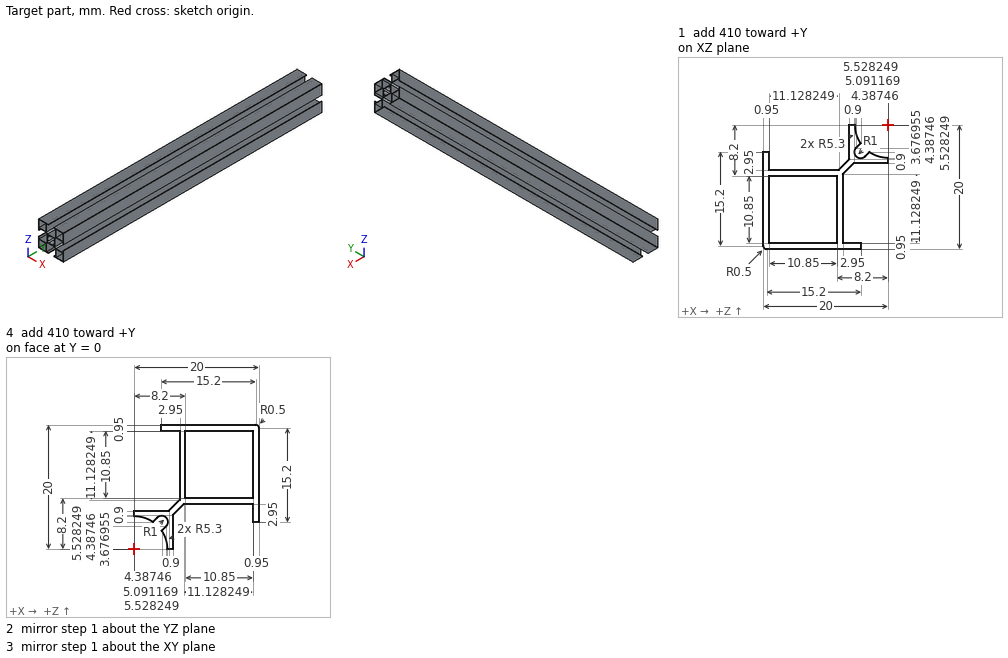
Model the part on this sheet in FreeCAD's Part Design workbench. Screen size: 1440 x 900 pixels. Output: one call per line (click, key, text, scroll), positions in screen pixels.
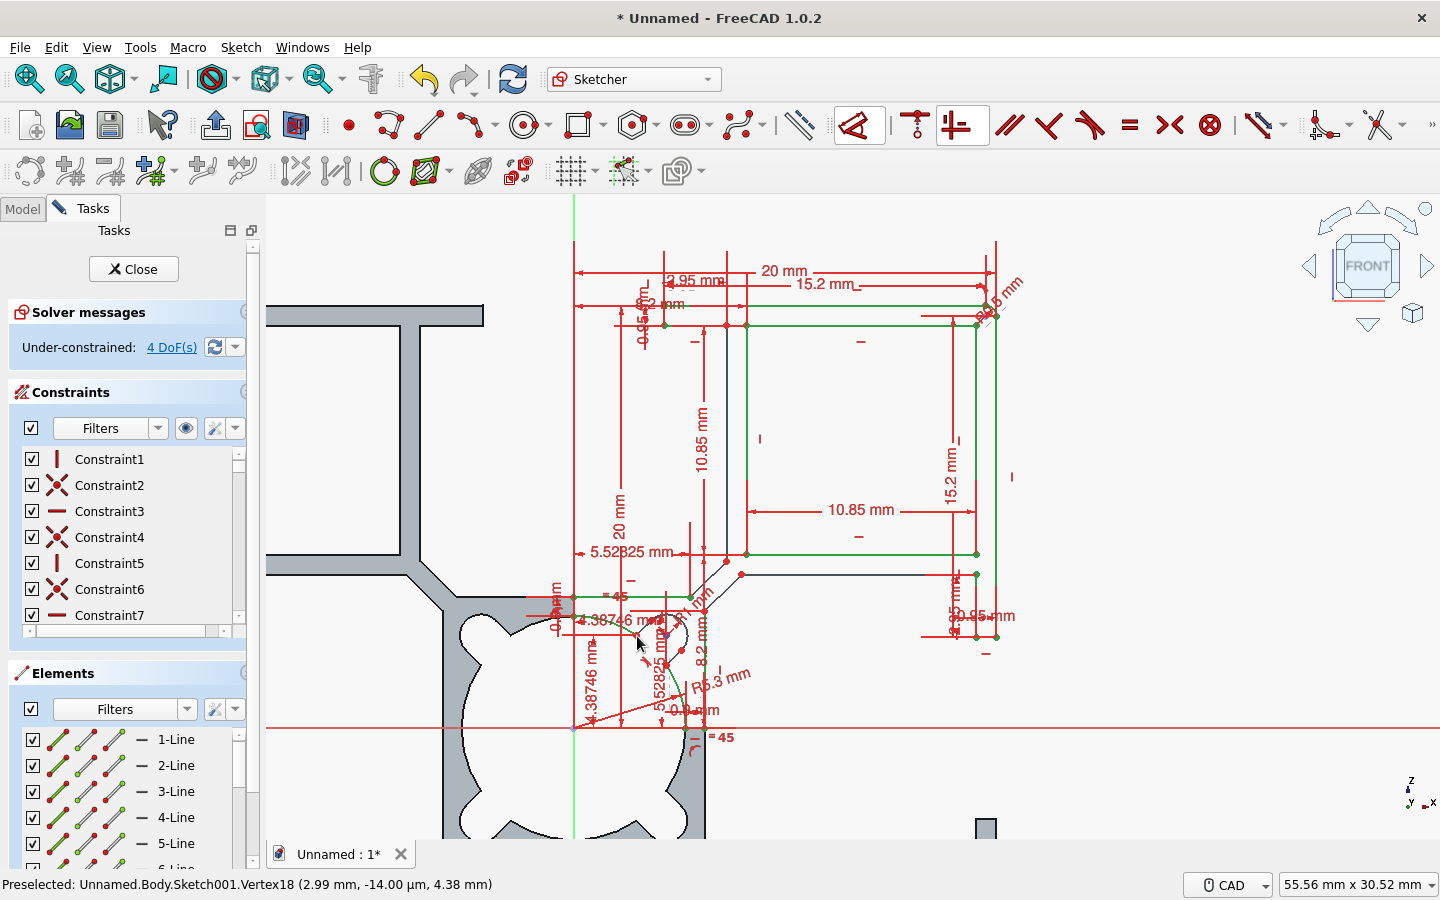
click(906, 575)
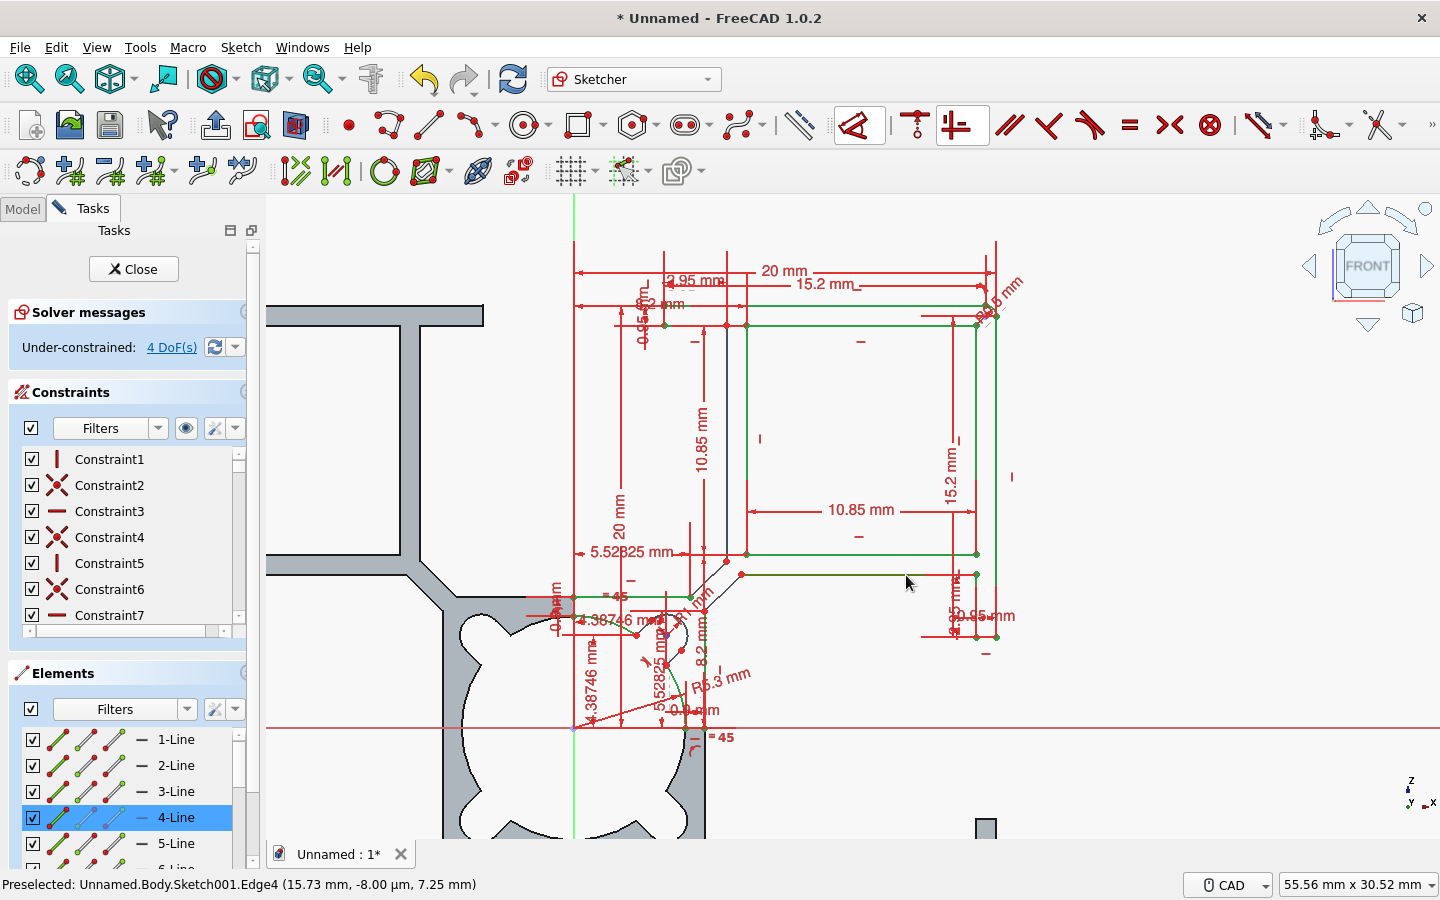
click(880, 126)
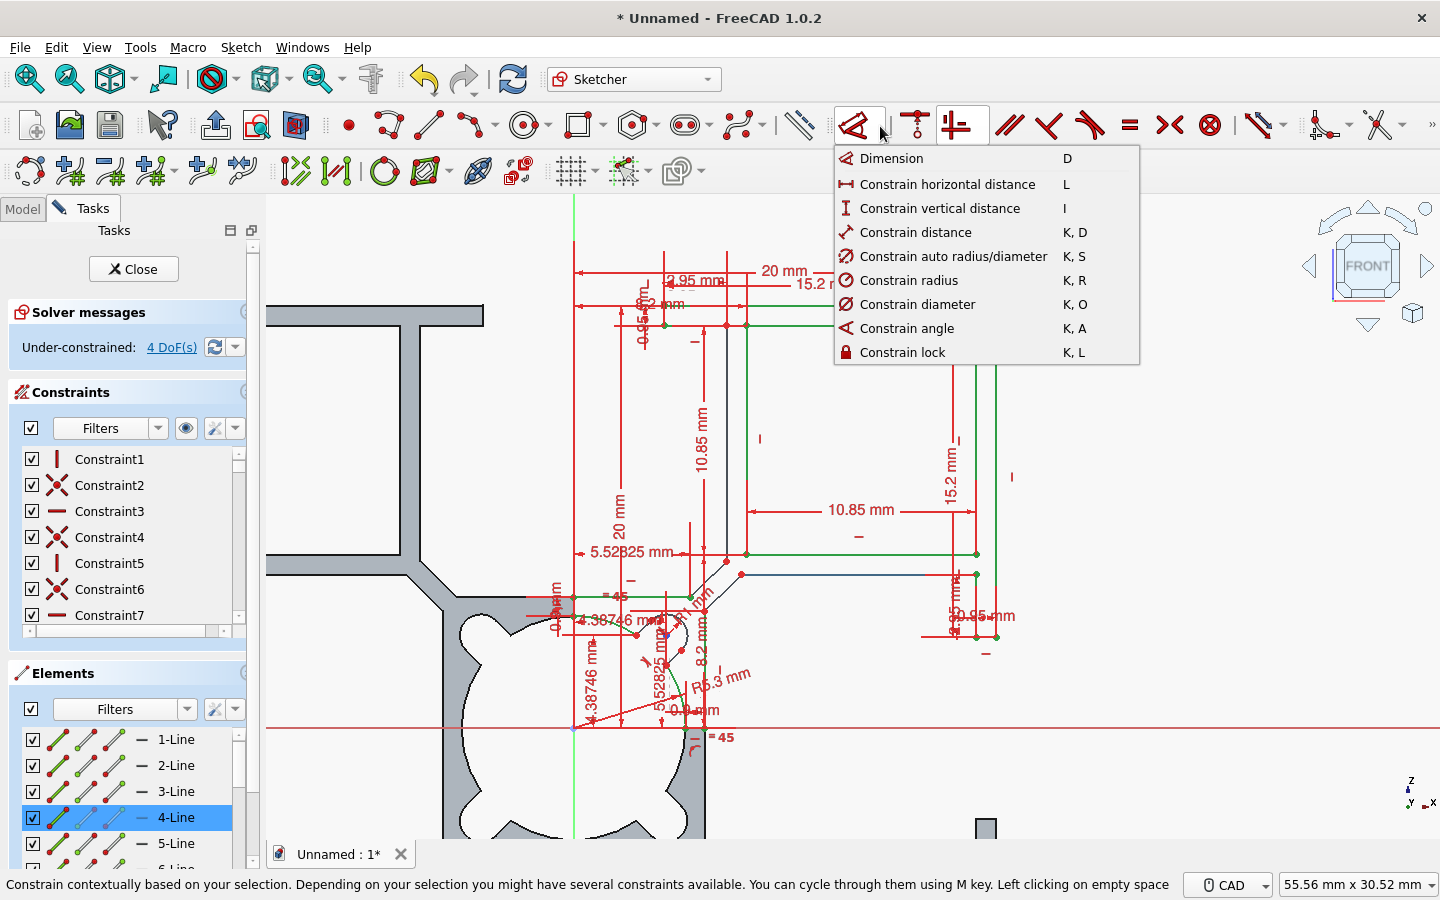
click(987, 184)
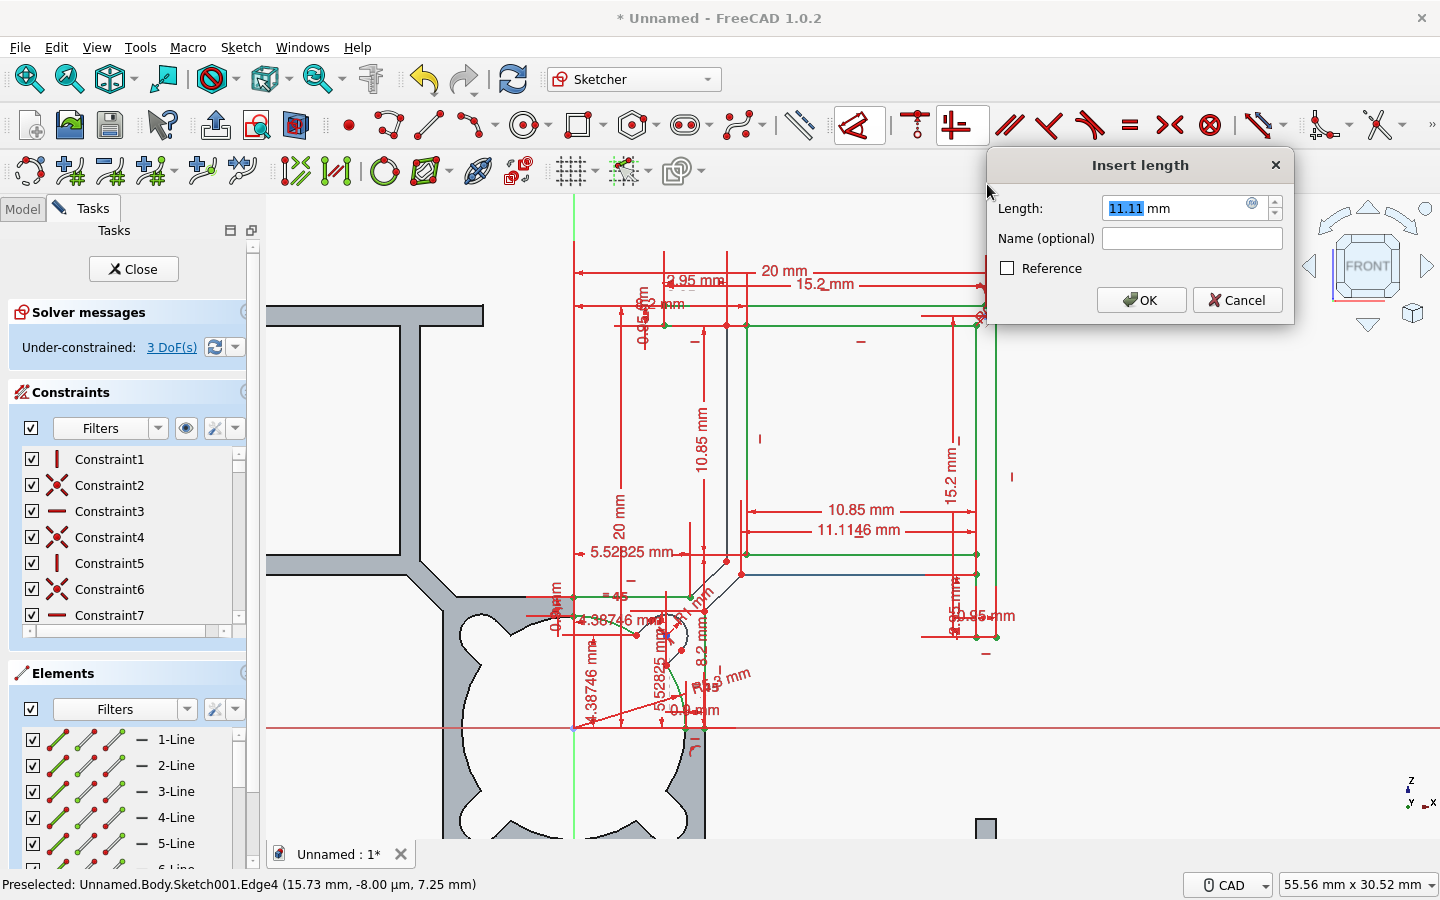
text(11.128249)
key(Return)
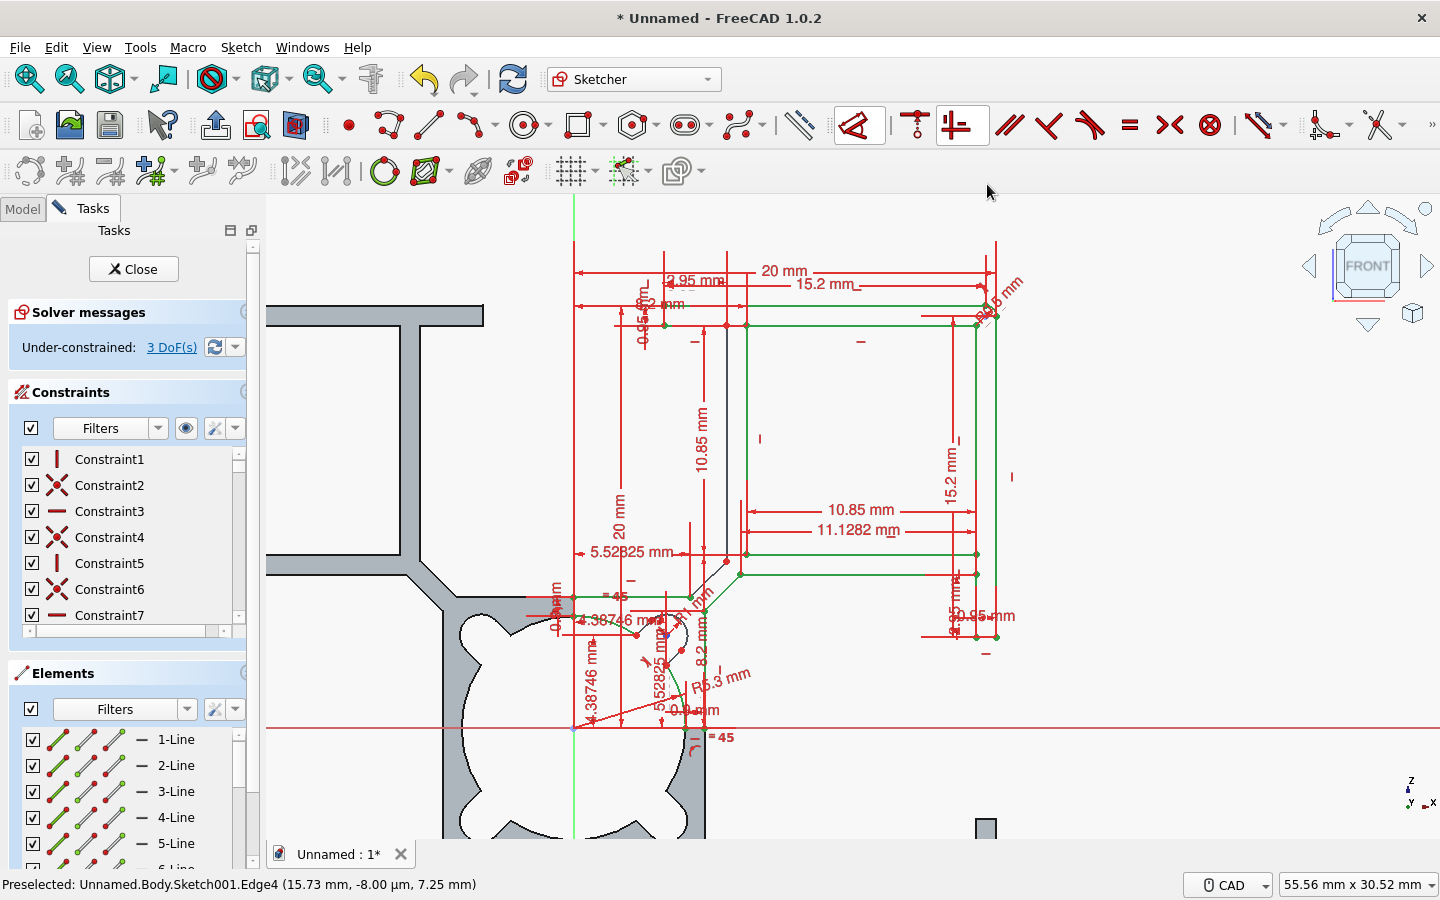
click(727, 491)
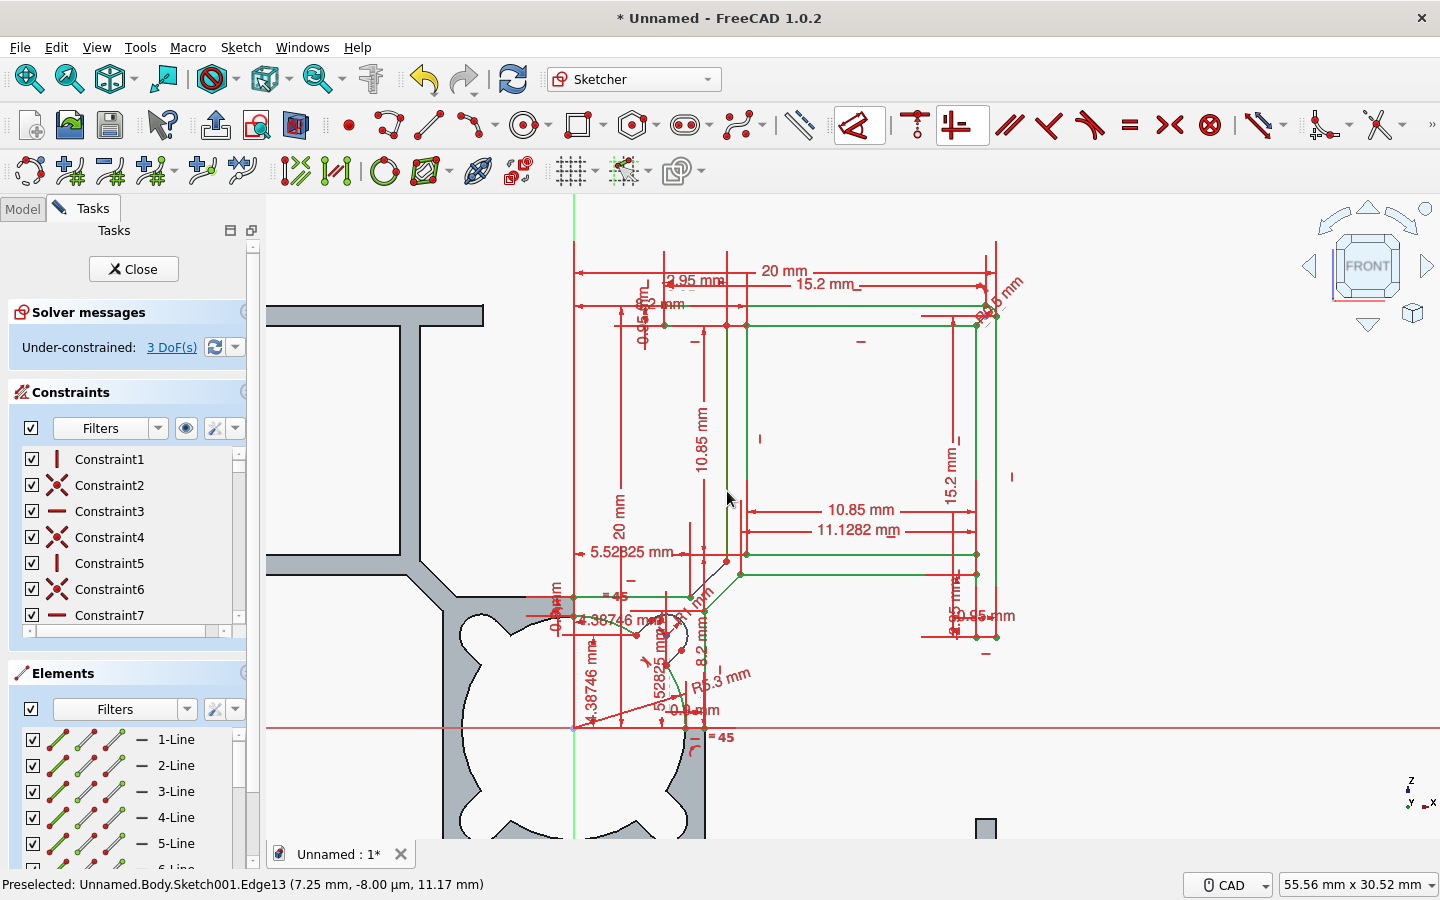
key(i)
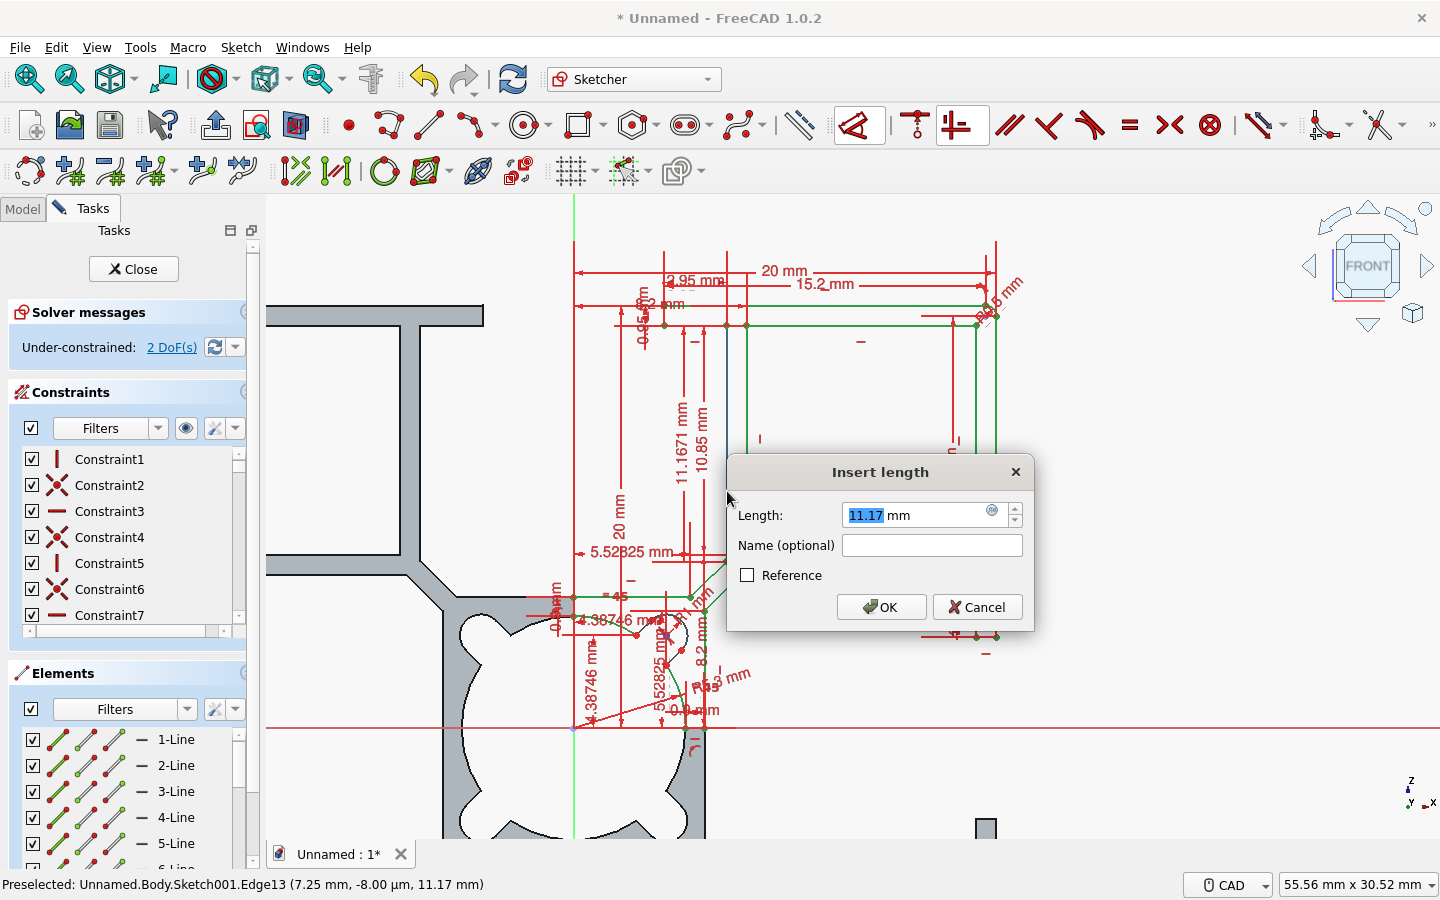
text(11.128249)
key(Return)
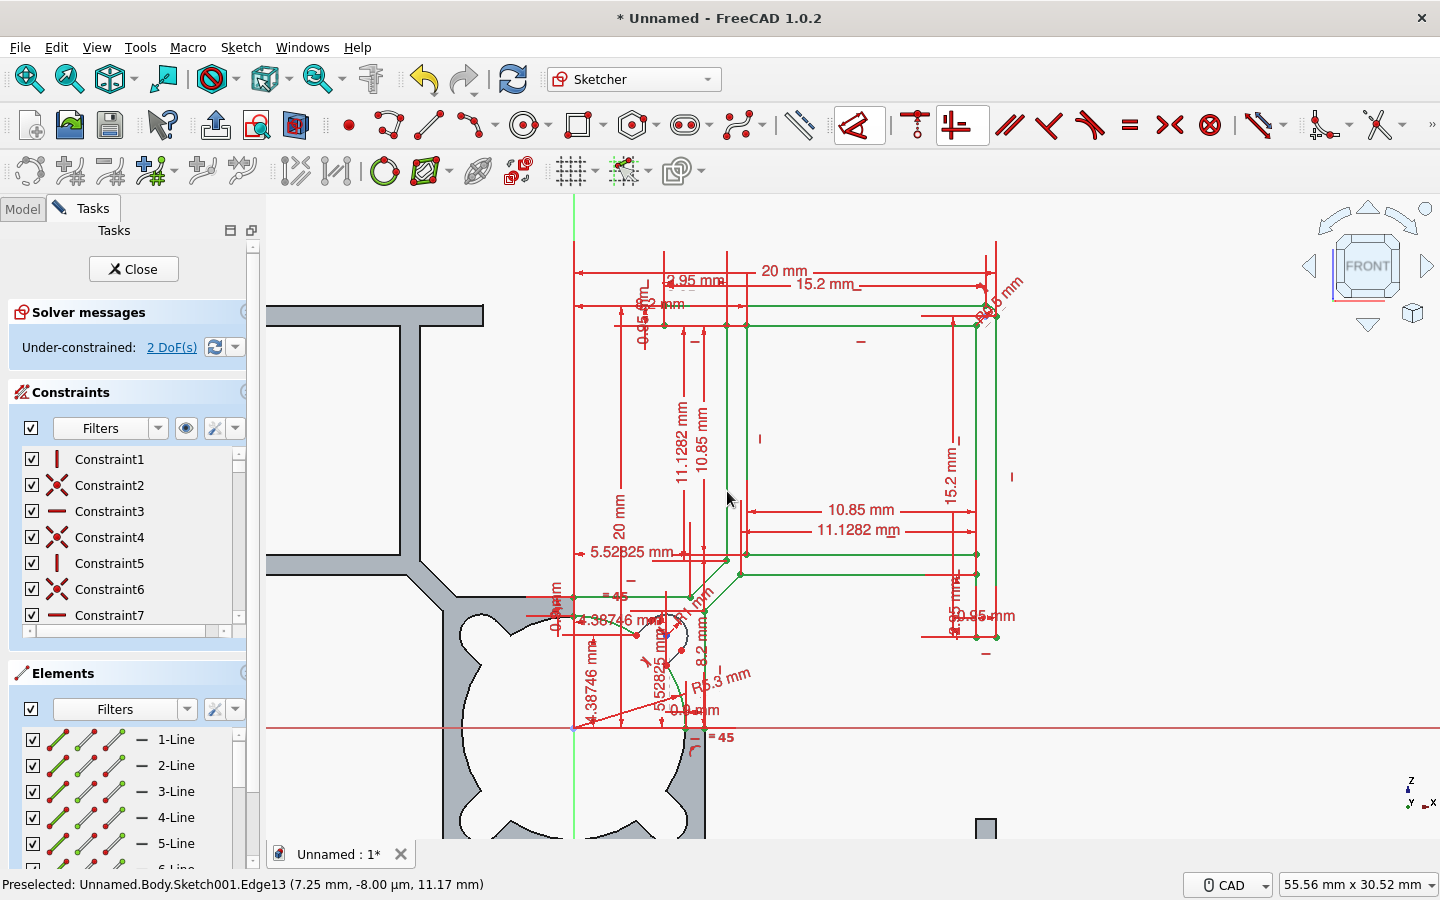
click(681, 651)